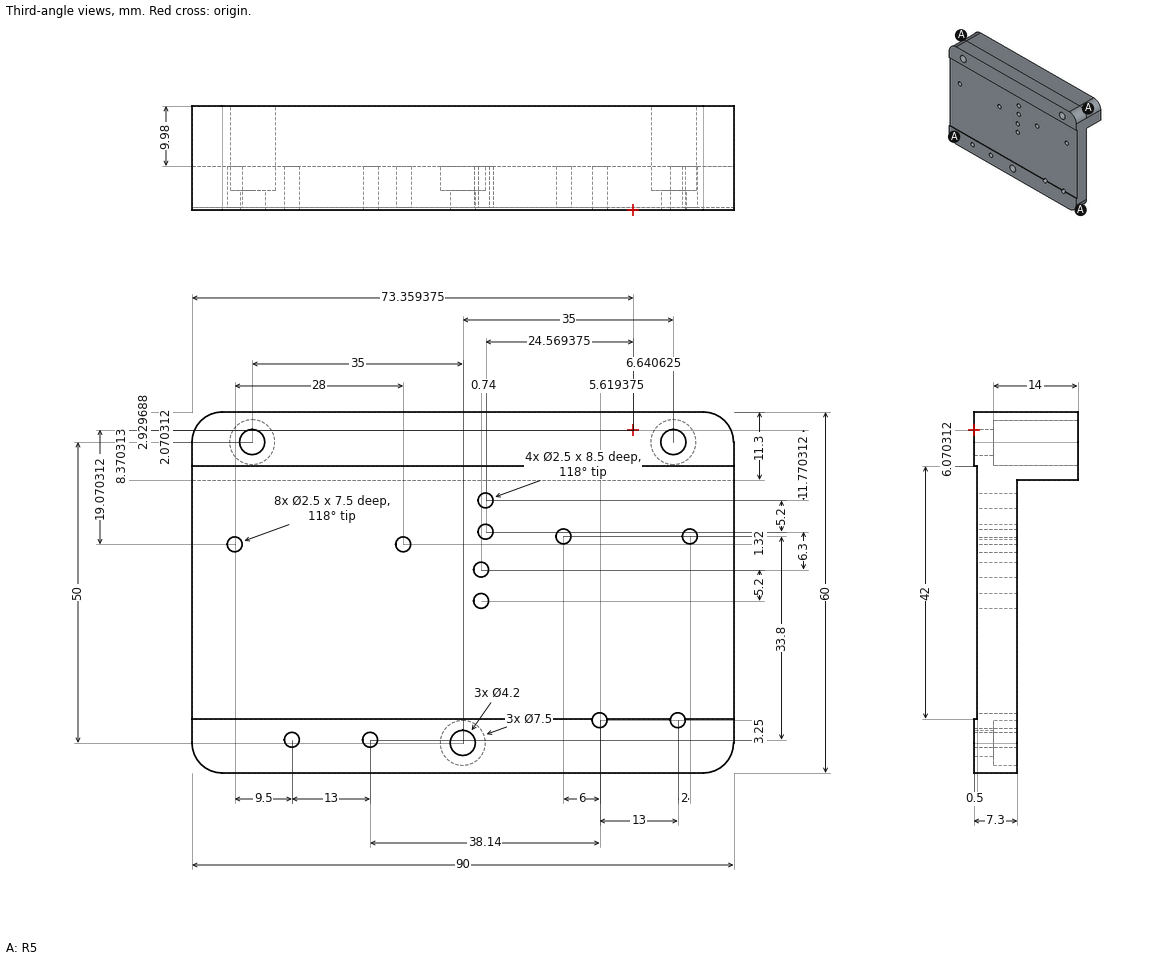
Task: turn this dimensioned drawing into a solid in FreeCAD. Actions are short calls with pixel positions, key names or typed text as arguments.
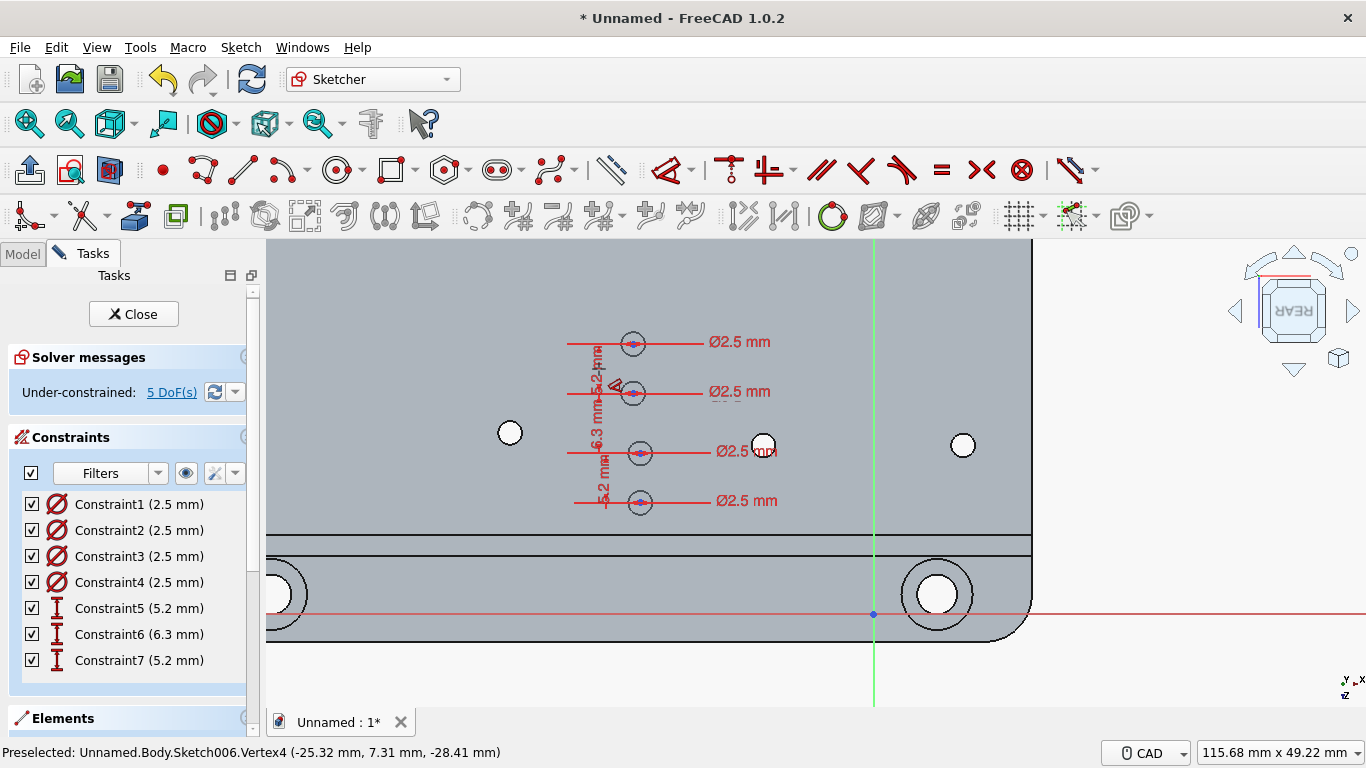
scroll(640, 453, up, 9)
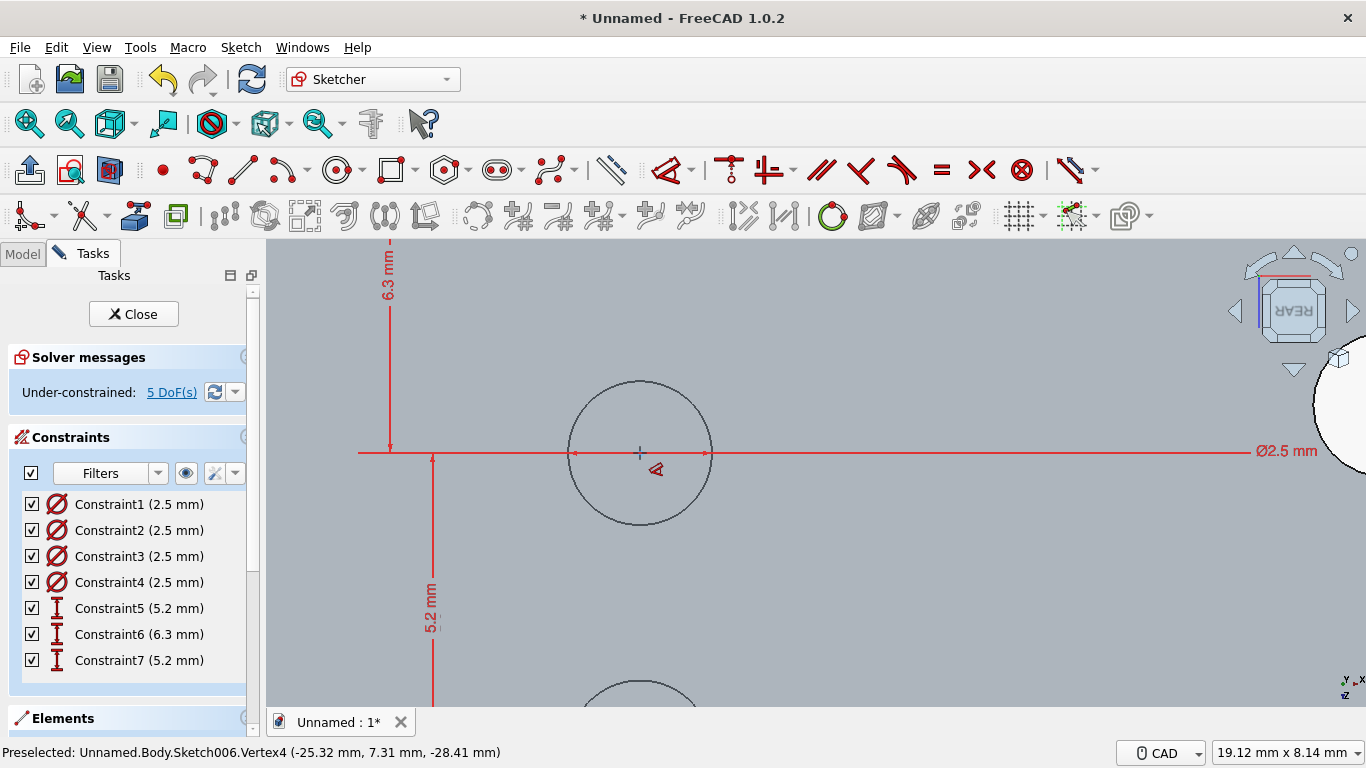
click(640, 453)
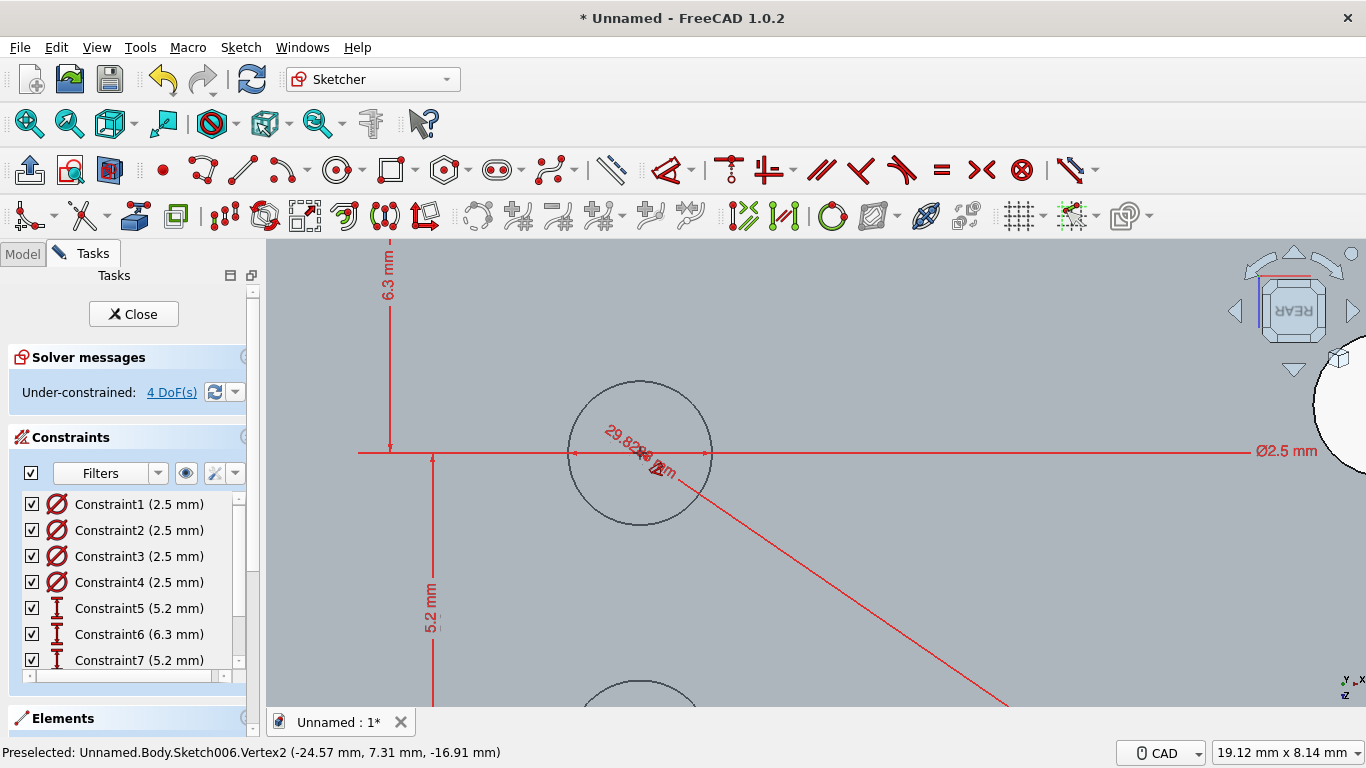
scroll(640, 454, down, 9)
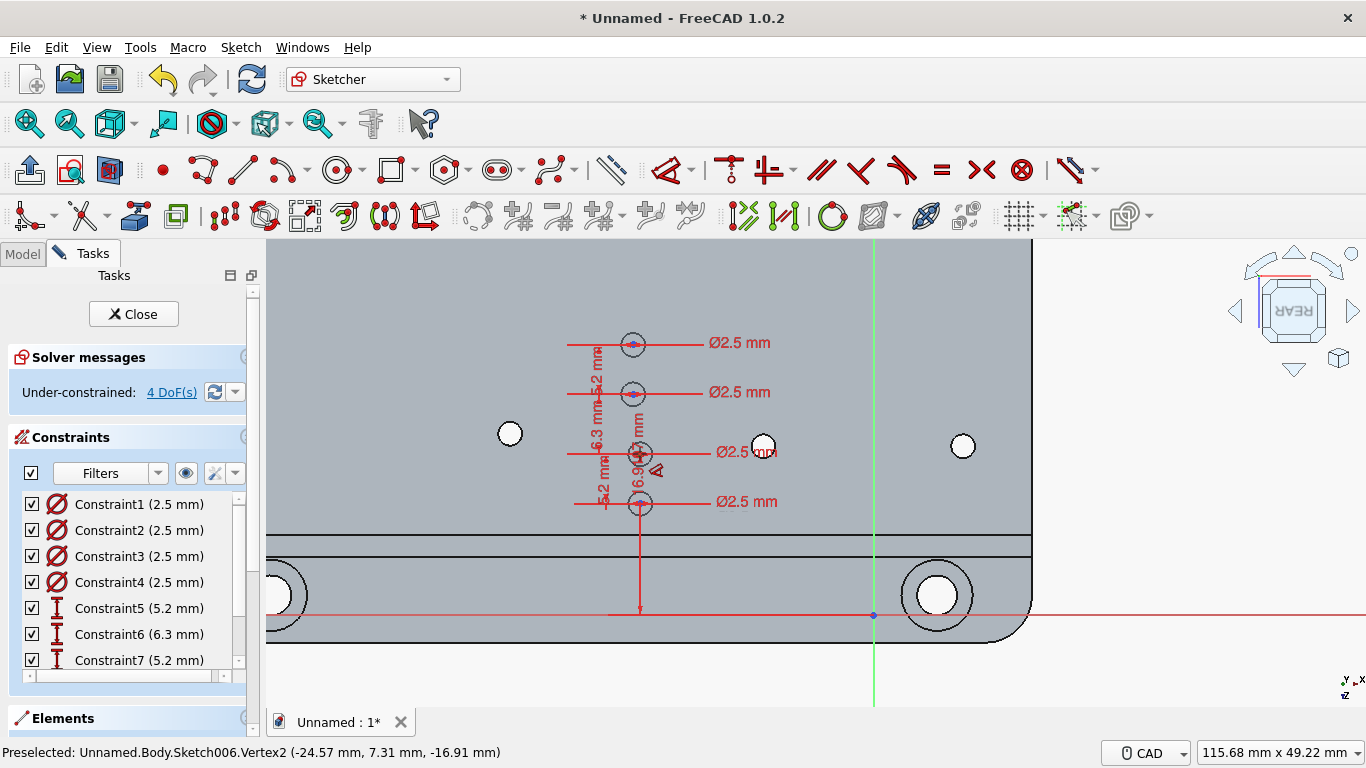
scroll(633, 394, up, 9)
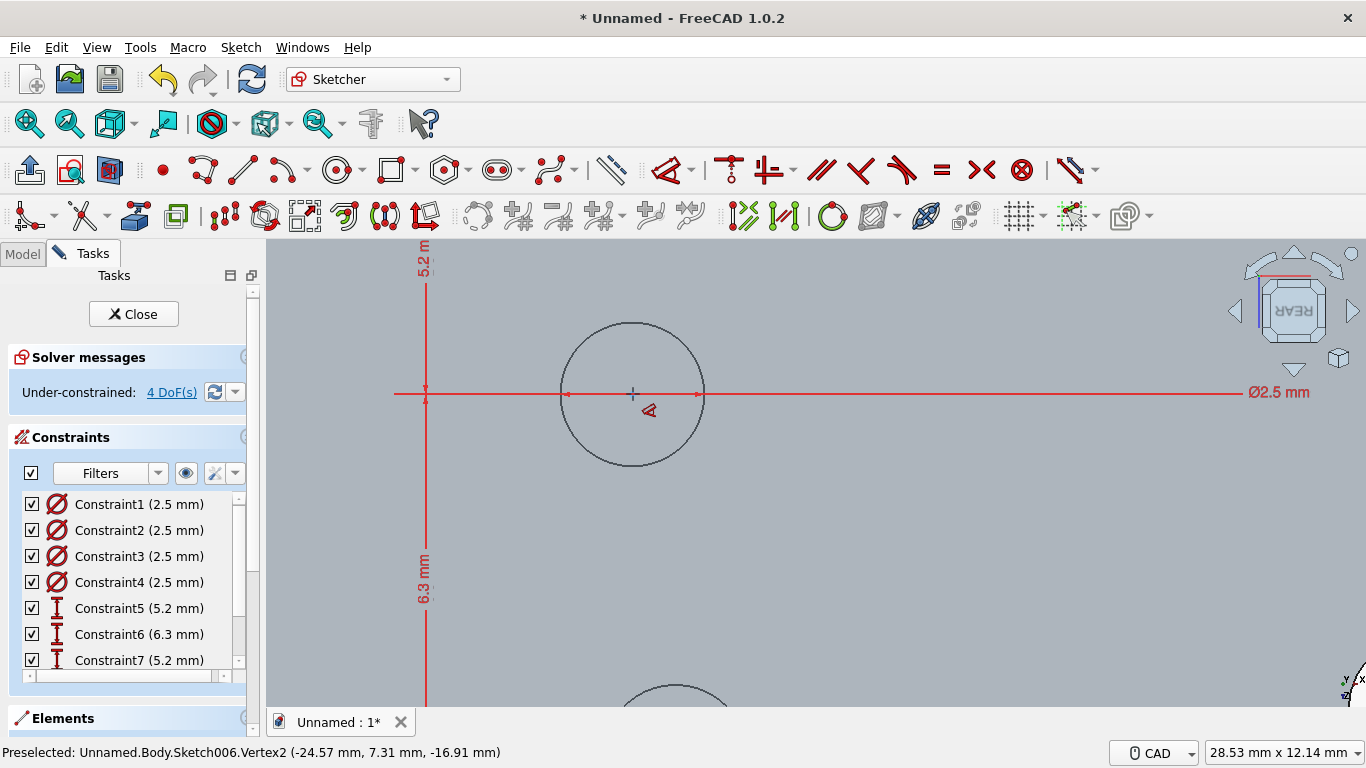
click(632, 394)
click(654, 360)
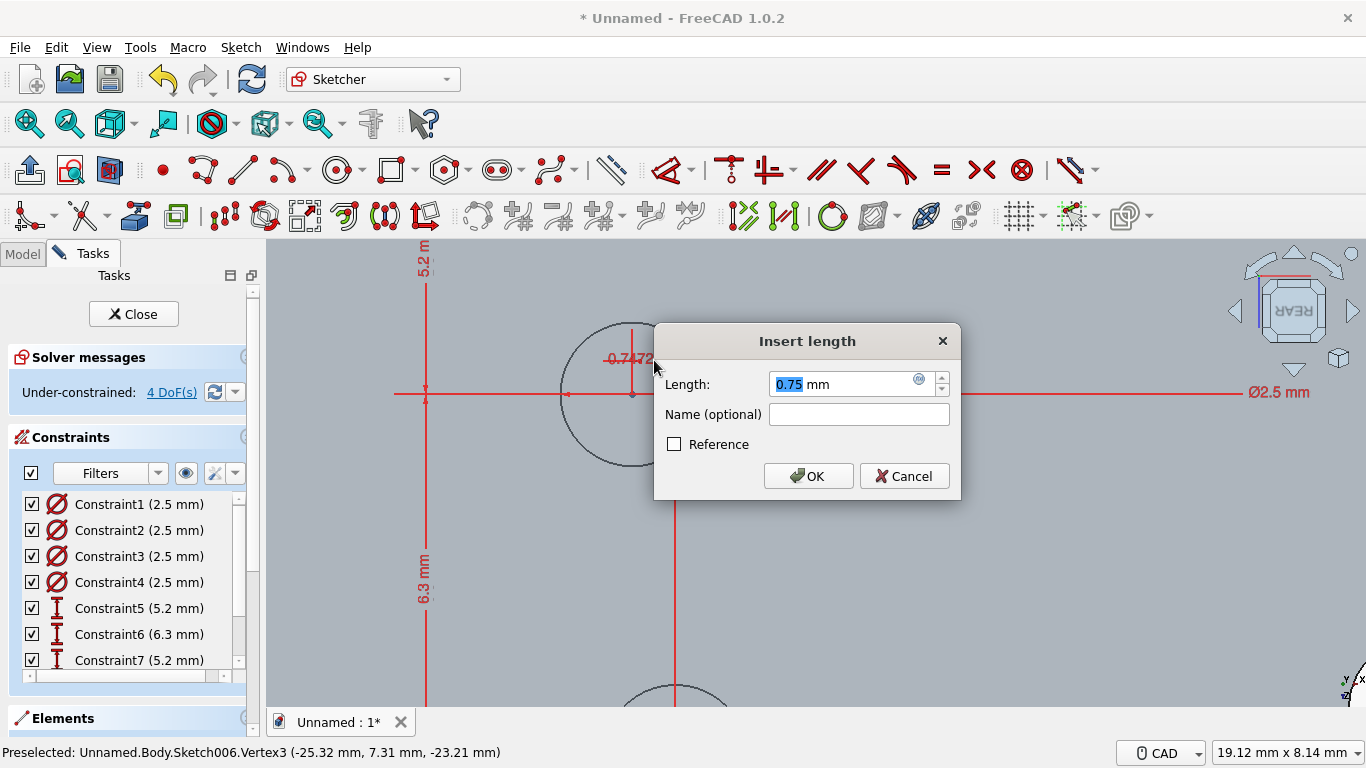
text(0.74)
key(Return)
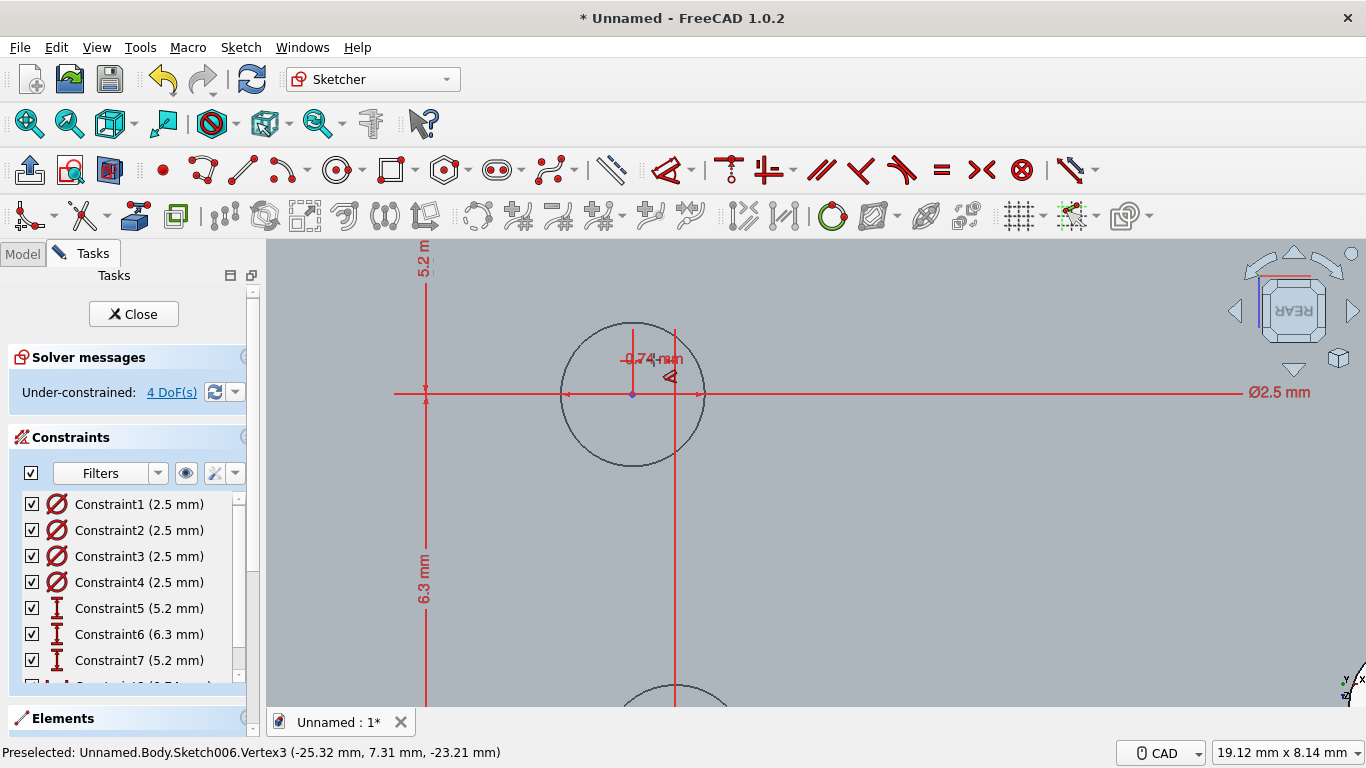
scroll(633, 393, down, 9)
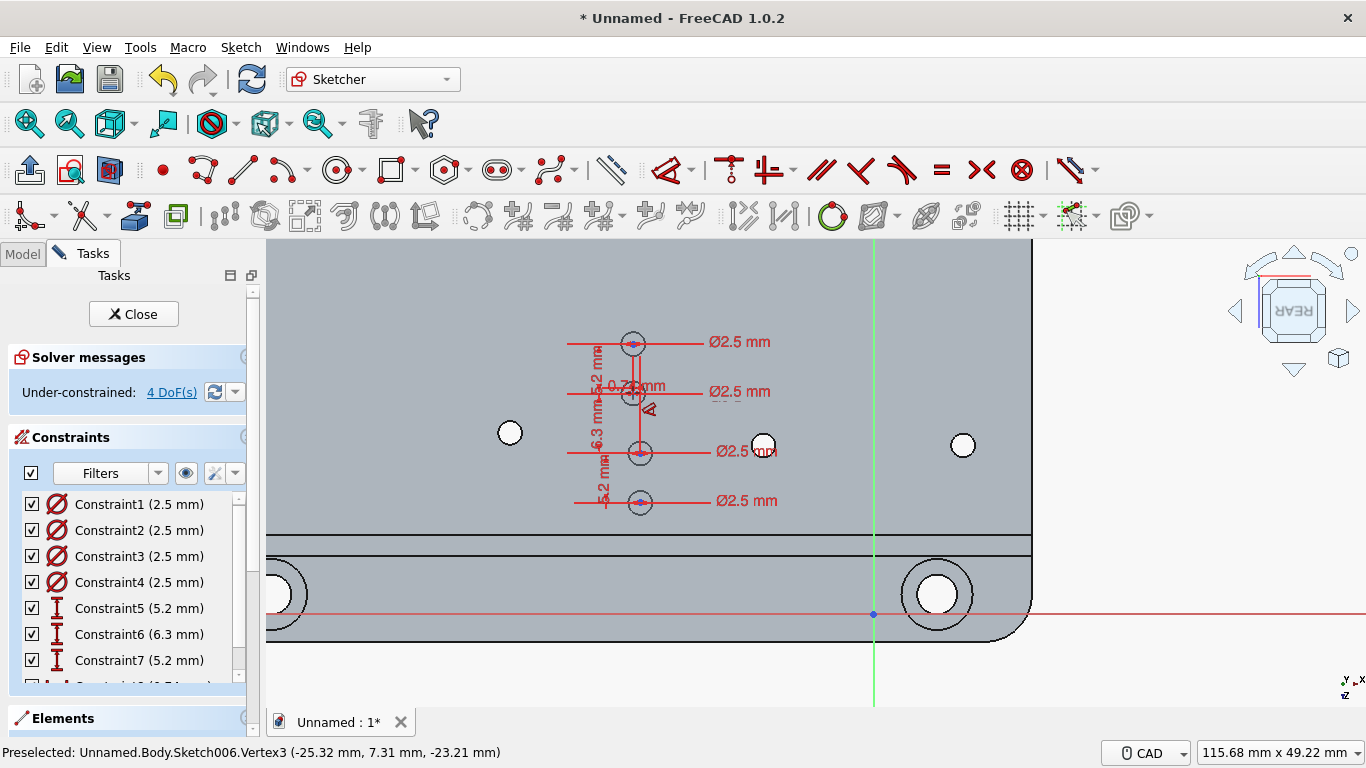
scroll(640, 503, up, 9)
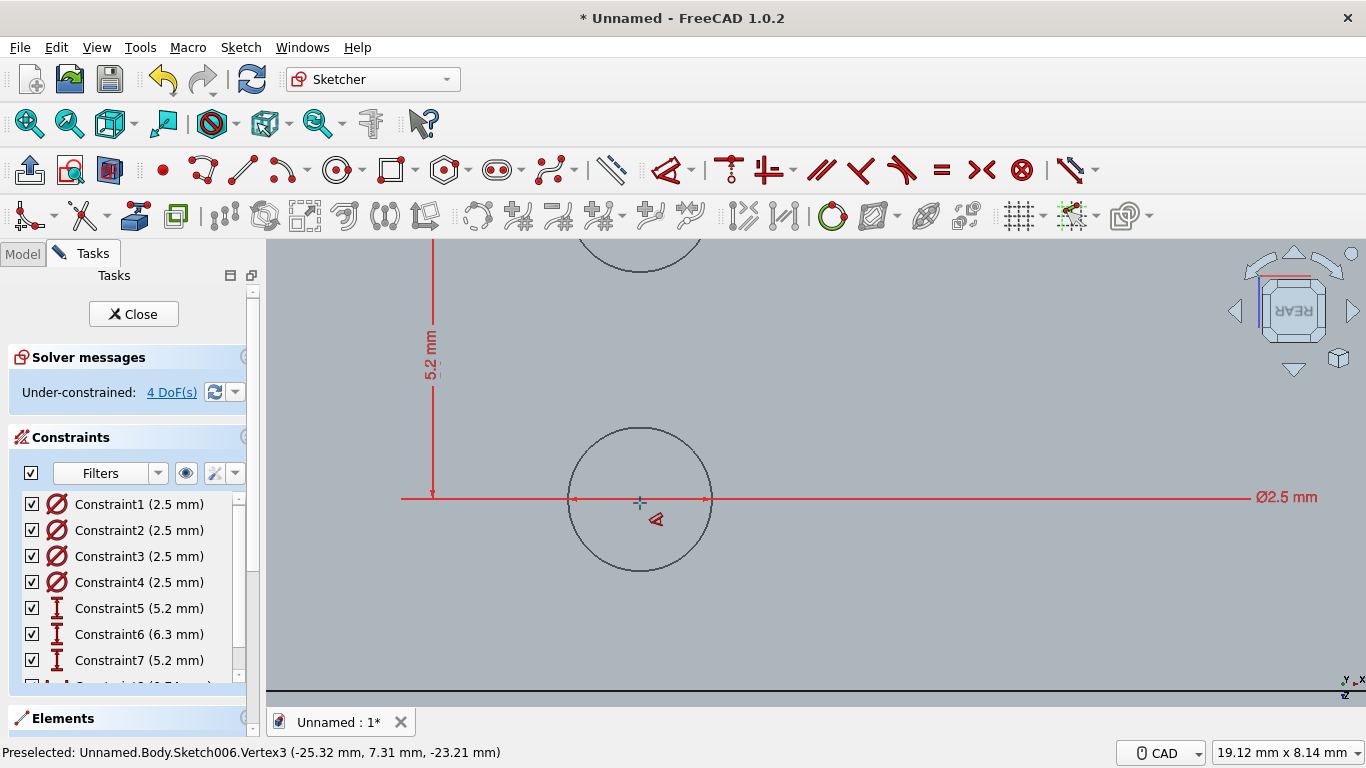
click(640, 499)